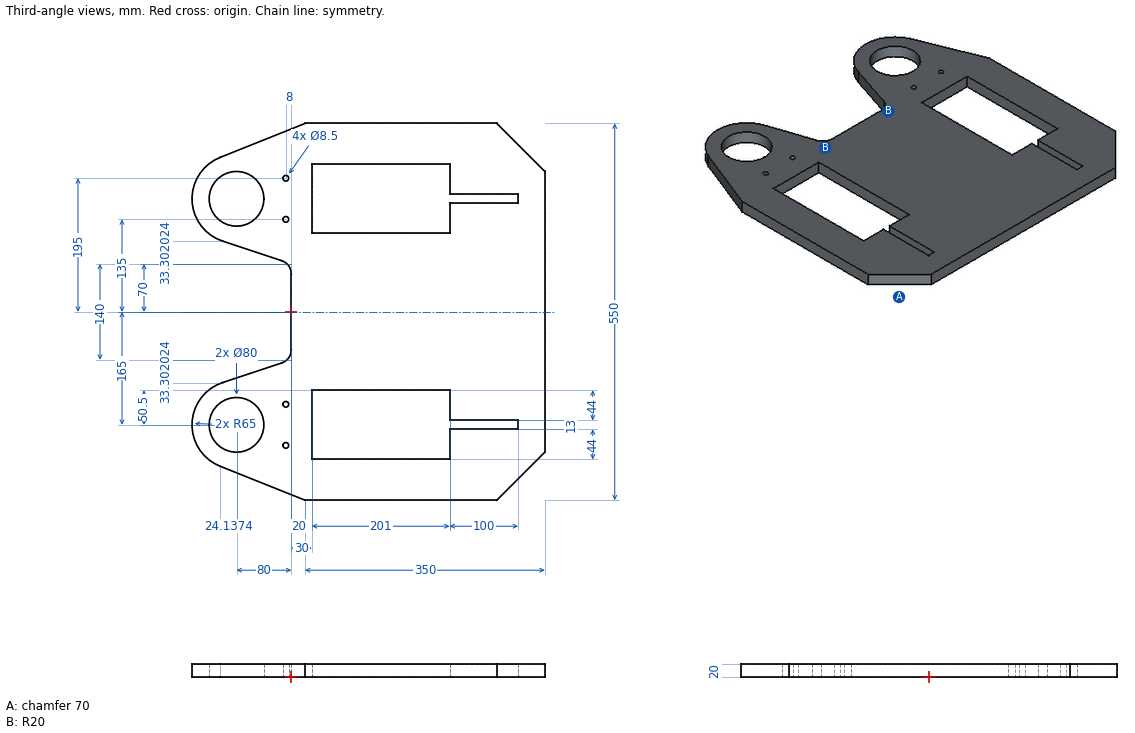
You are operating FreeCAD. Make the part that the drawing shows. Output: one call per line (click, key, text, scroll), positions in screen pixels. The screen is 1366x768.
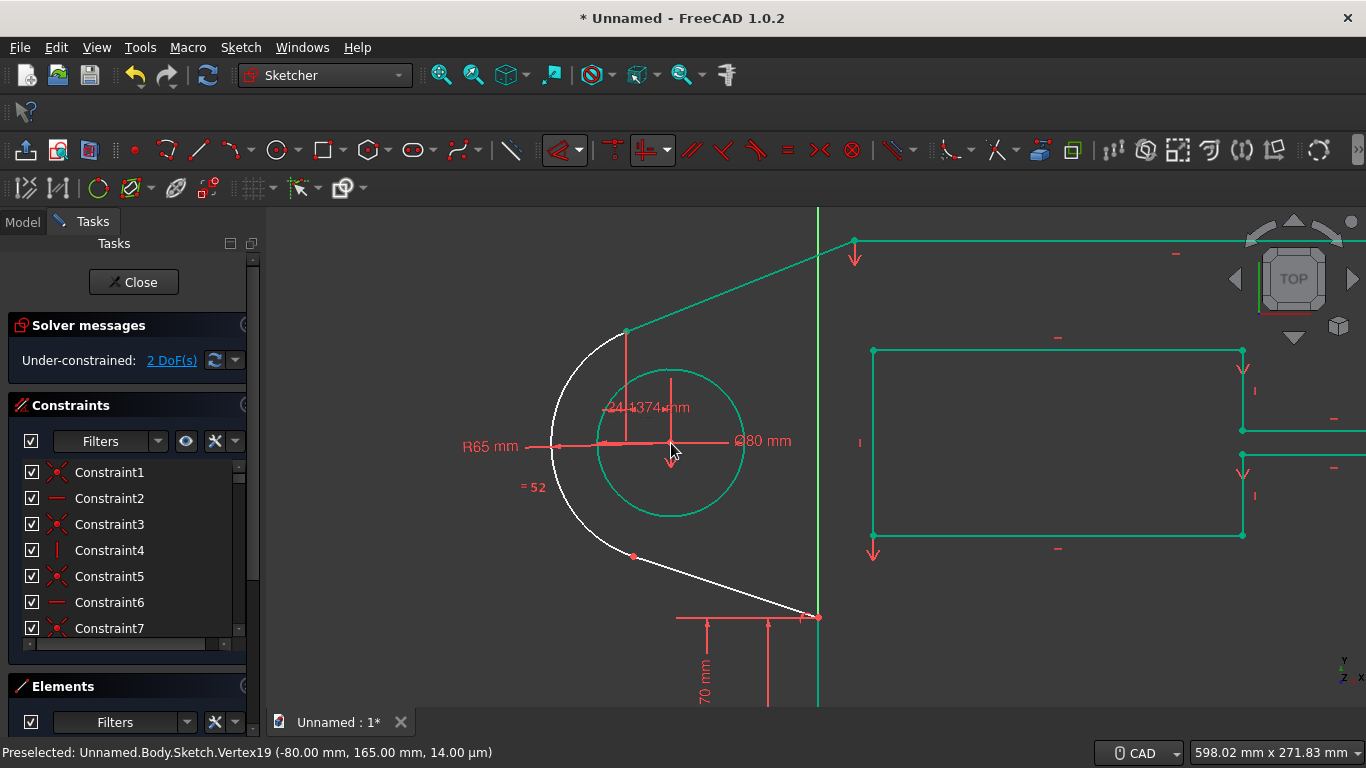
click(689, 575)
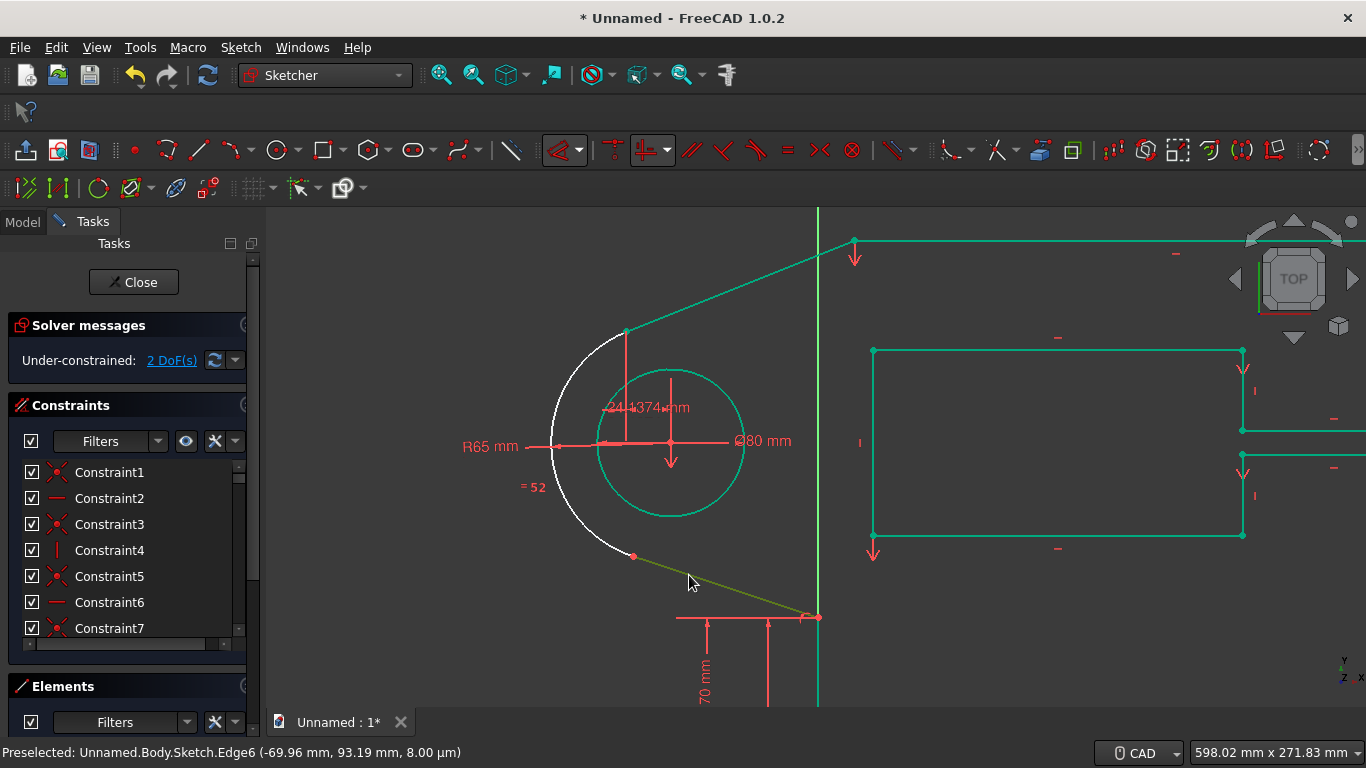
key(i)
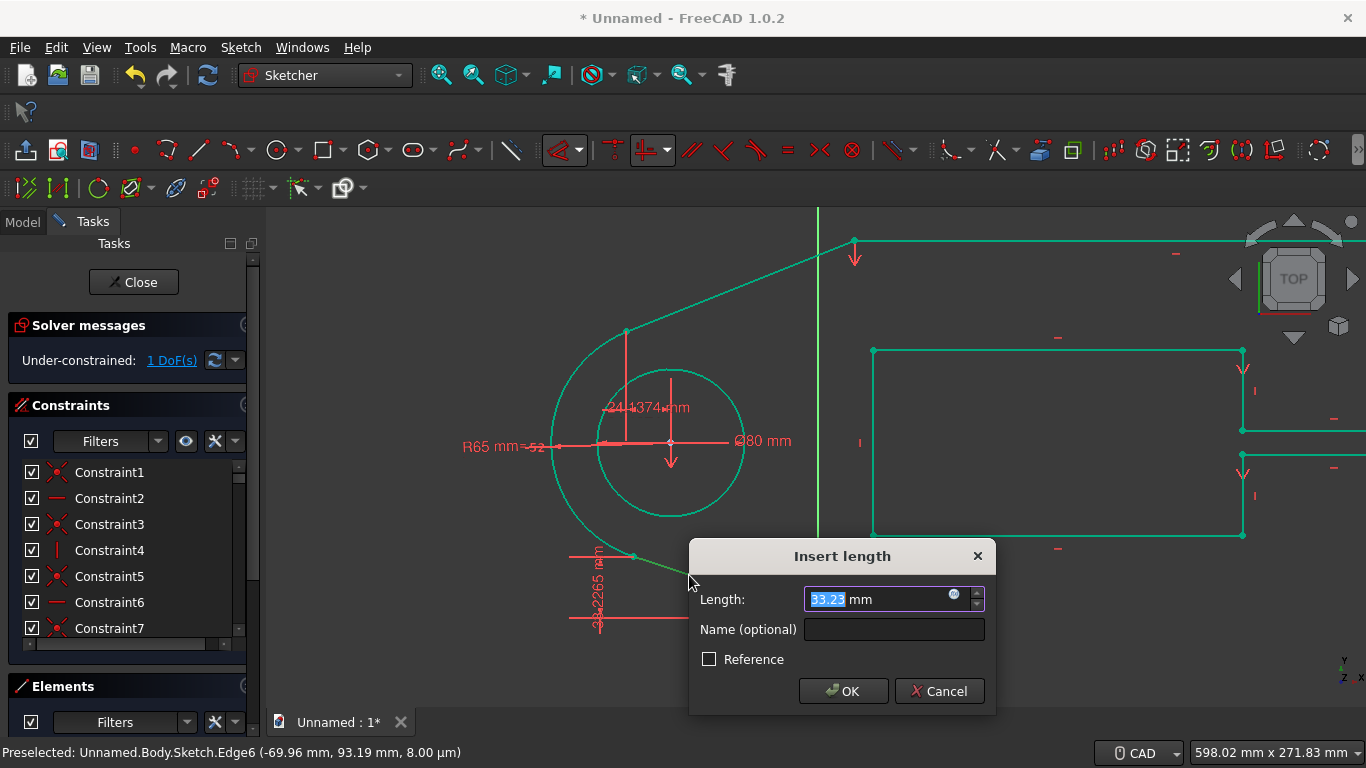
text(33.302024)
key(Return)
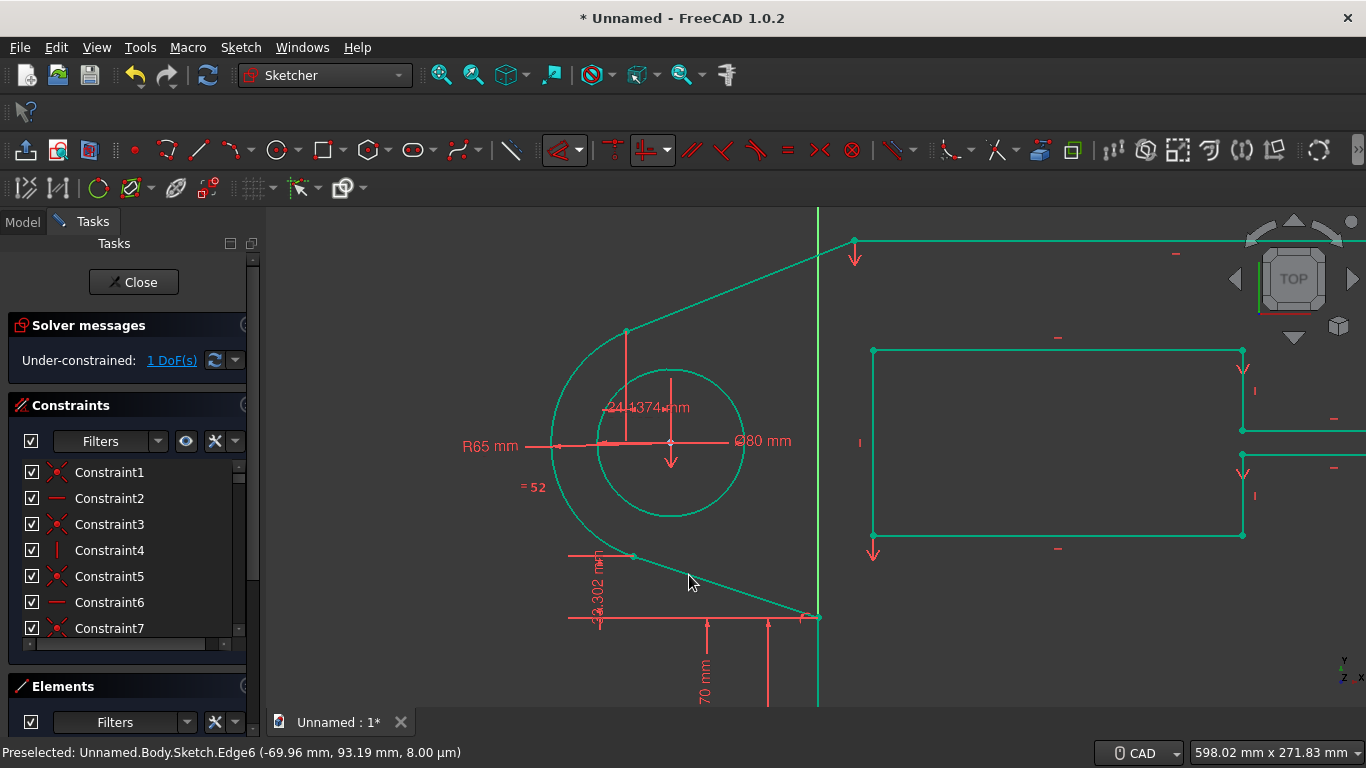
scroll(628, 332, down, 6)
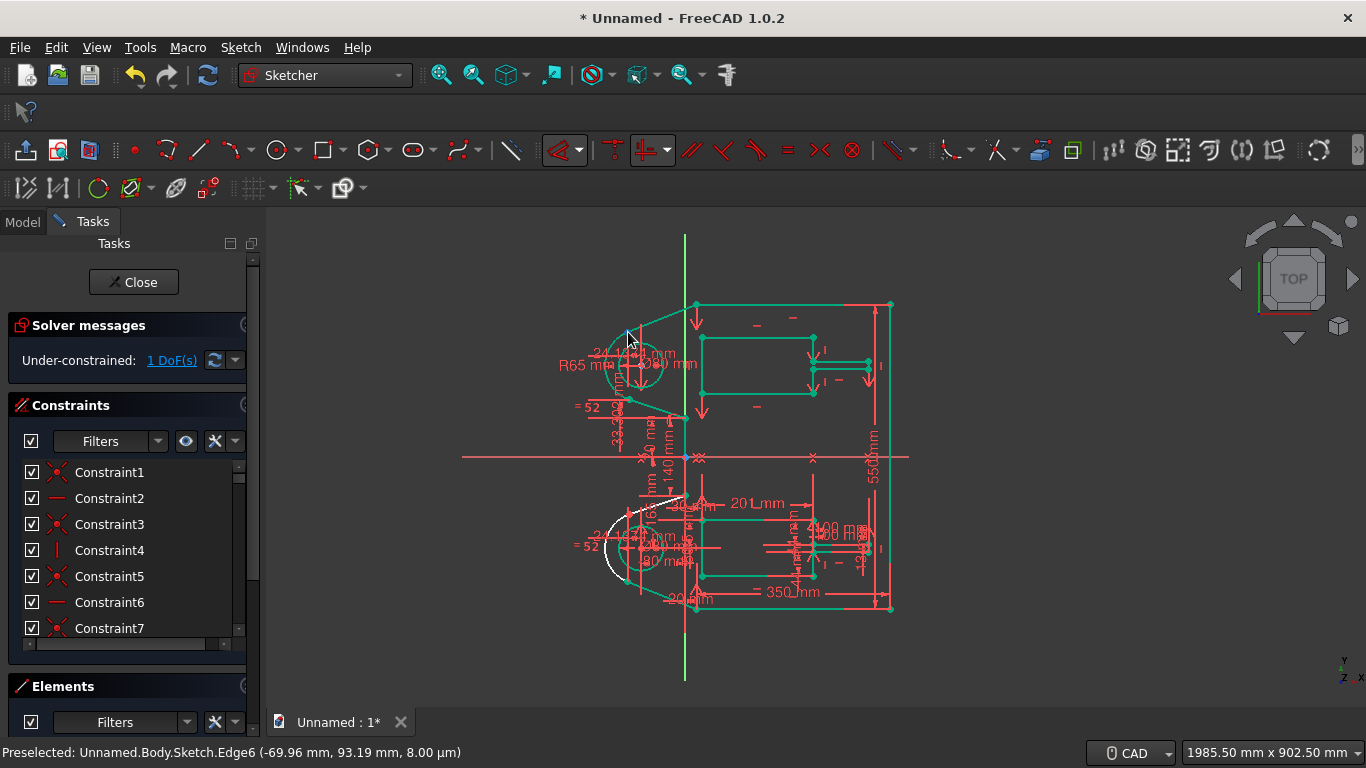
scroll(669, 501, up, 4)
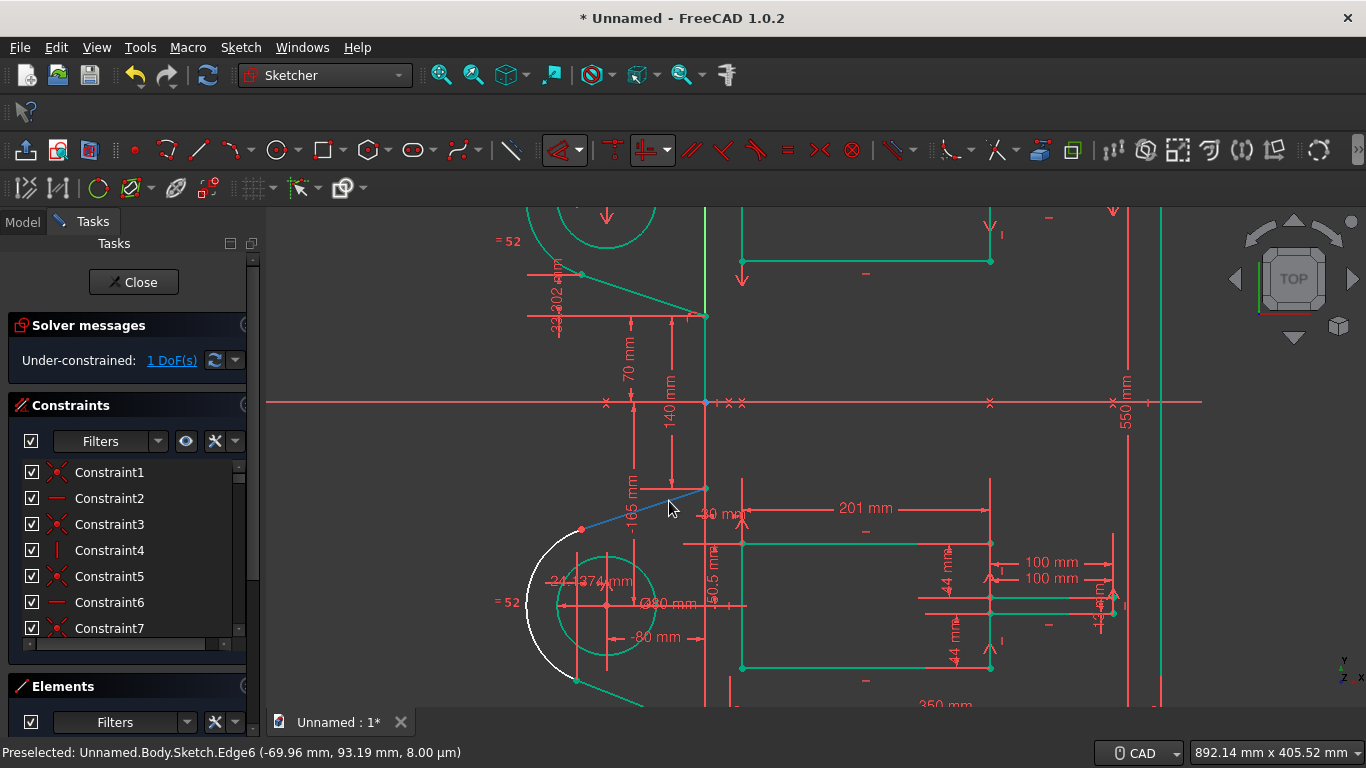
click(668, 501)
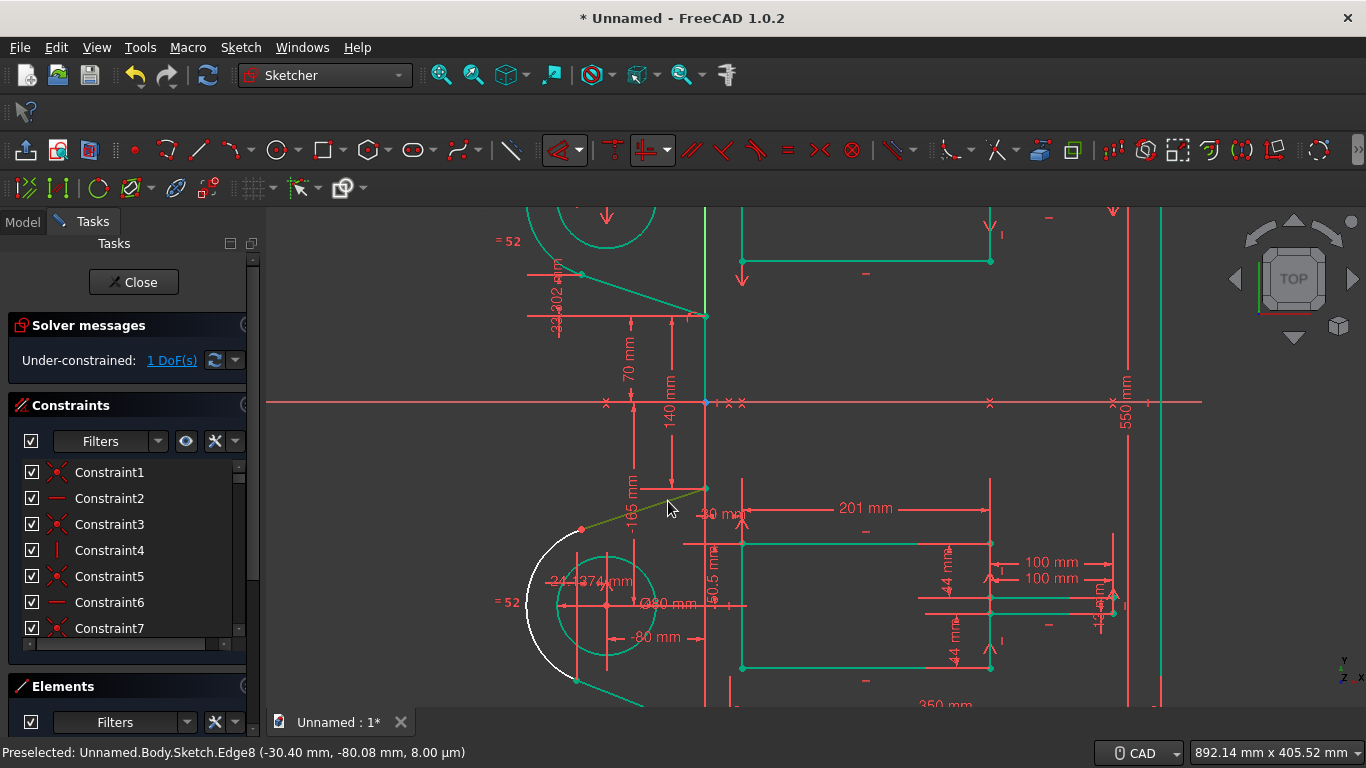
key(i)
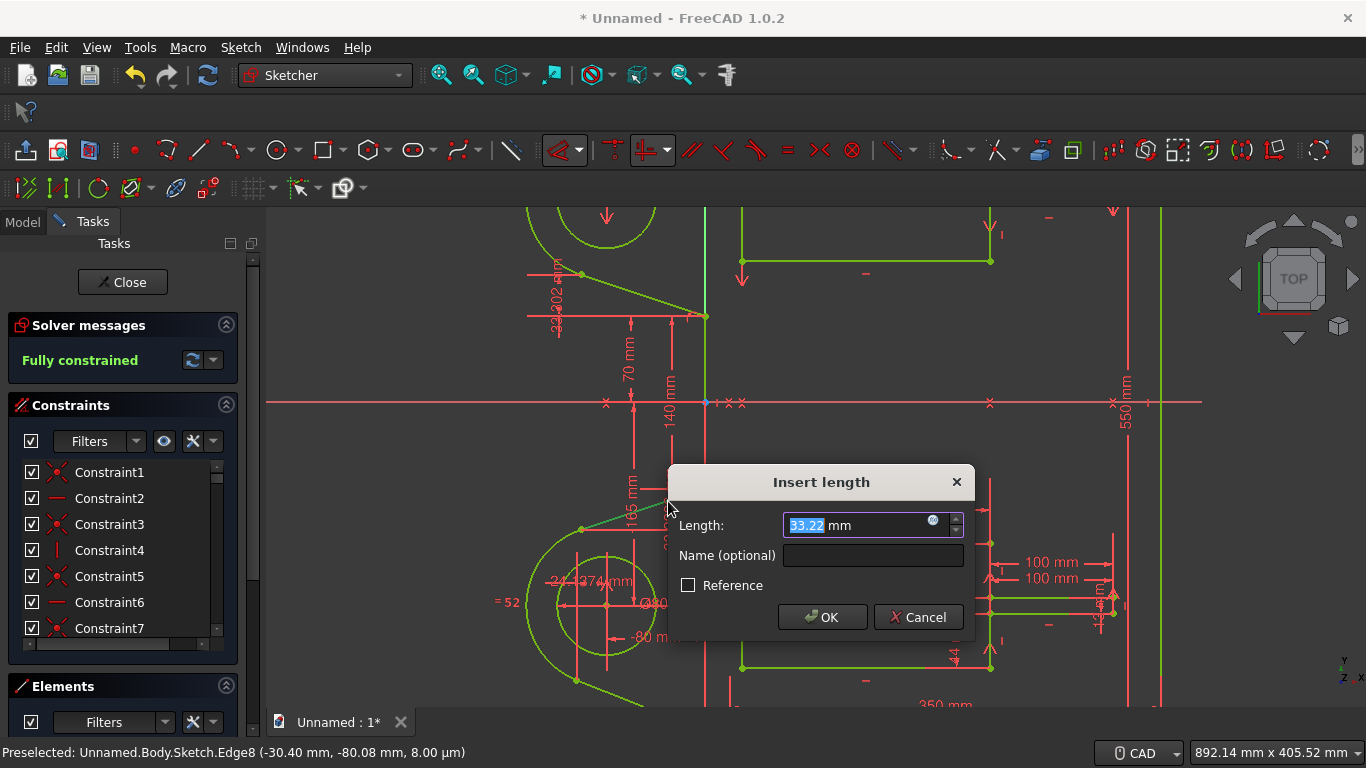
text(33.302024)
key(Return)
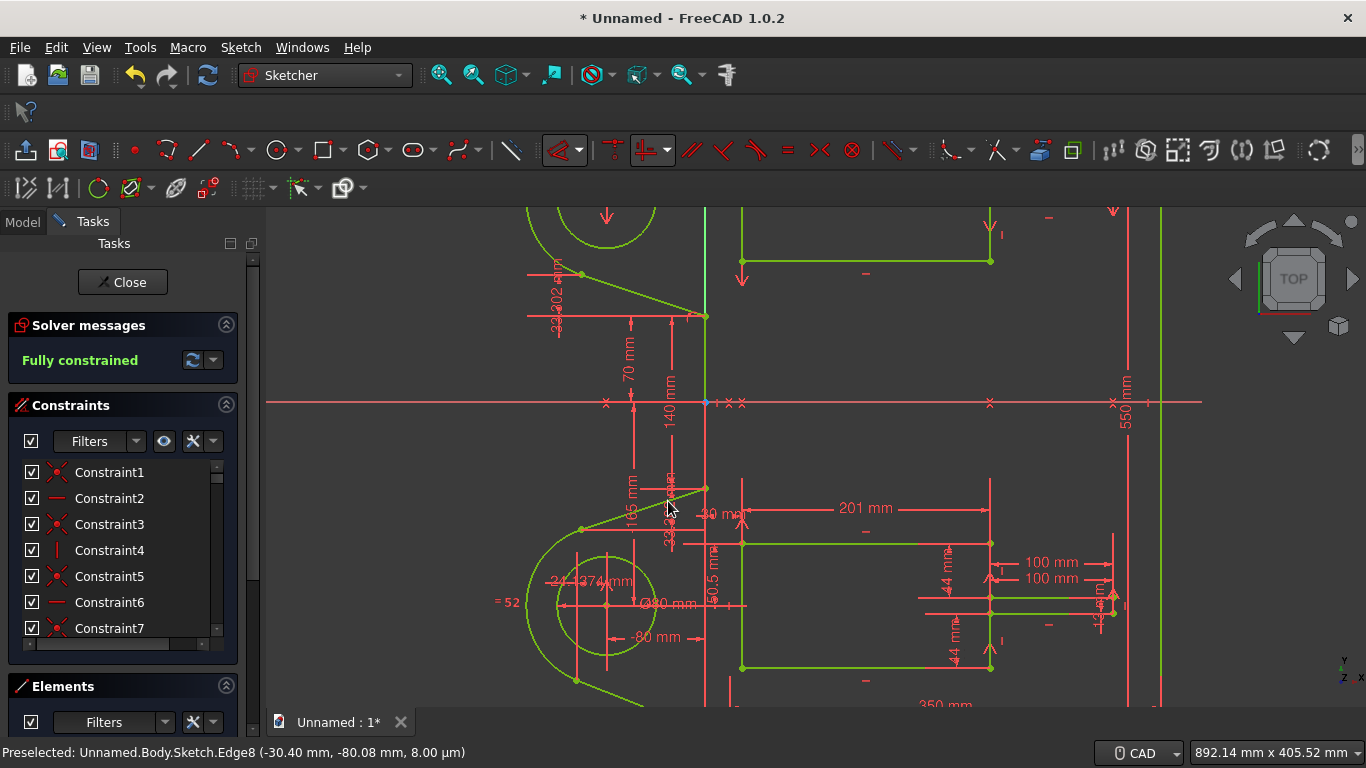
click(123, 282)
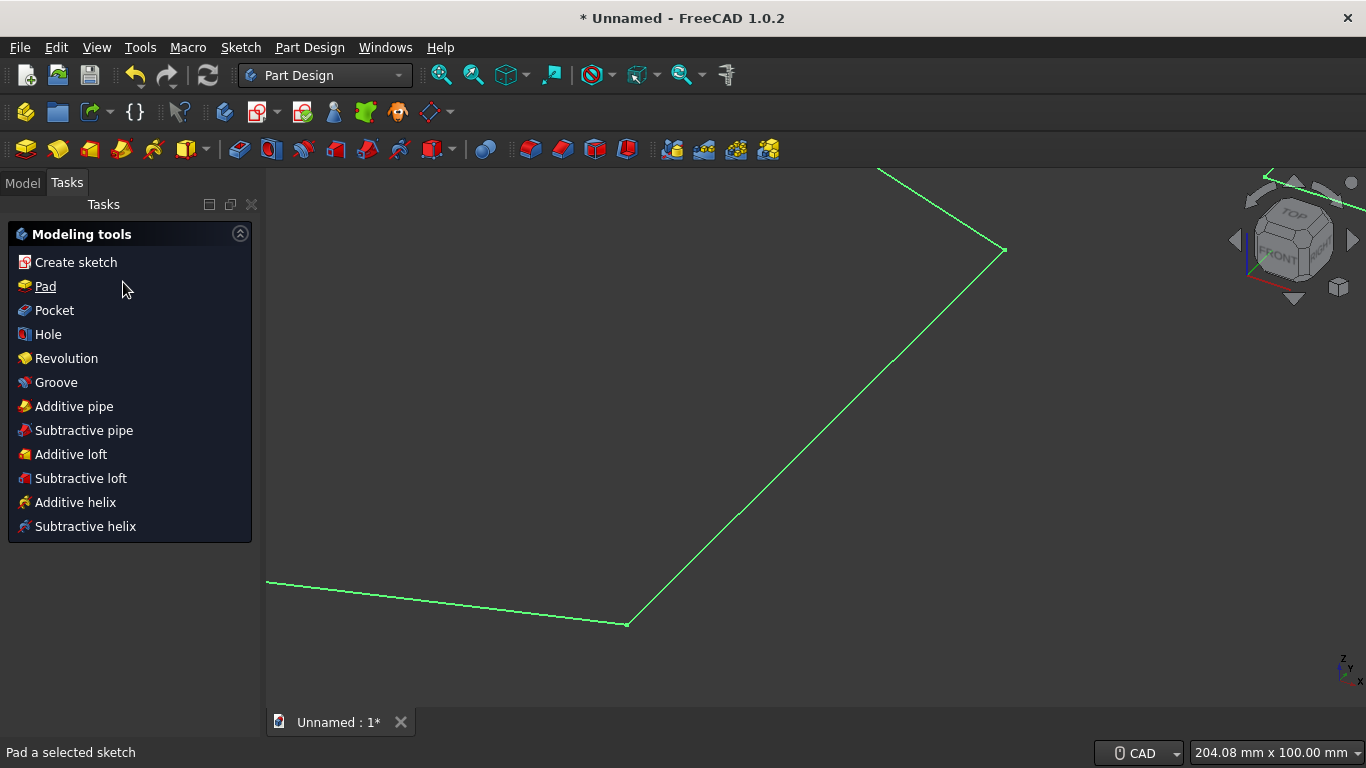
click(26, 150)